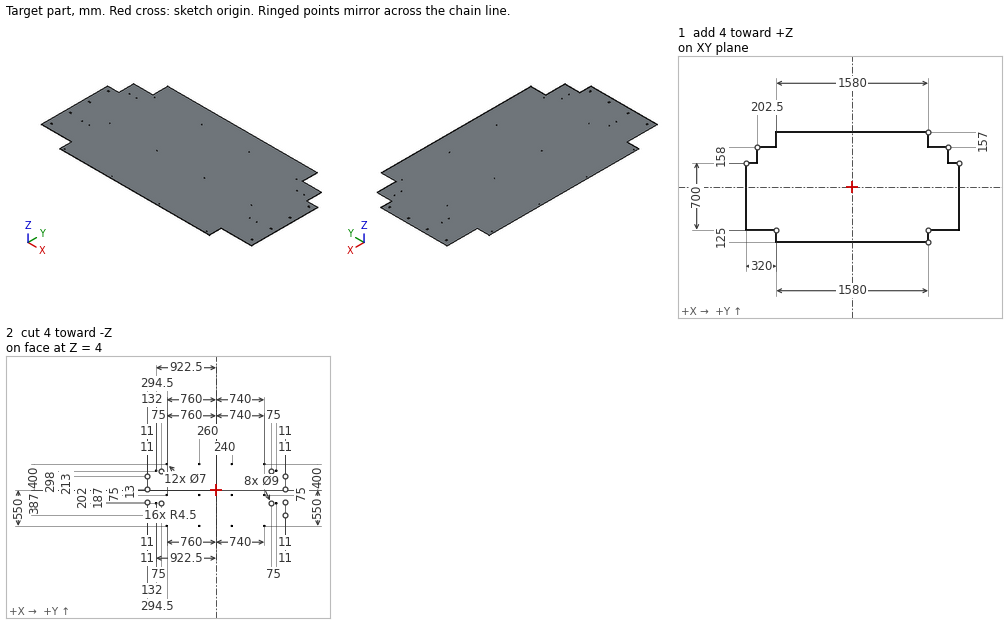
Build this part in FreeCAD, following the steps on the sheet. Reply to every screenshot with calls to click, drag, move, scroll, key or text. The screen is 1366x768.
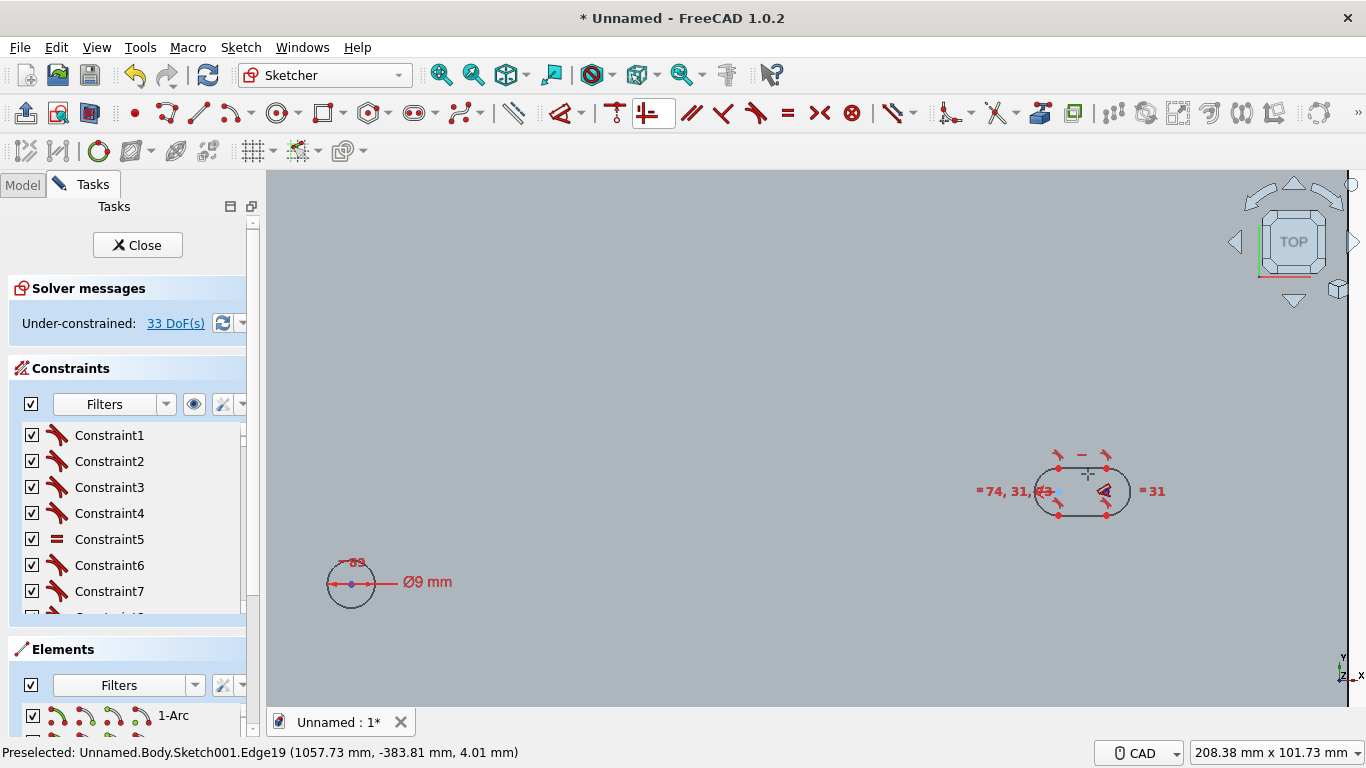
click(1073, 468)
click(1083, 502)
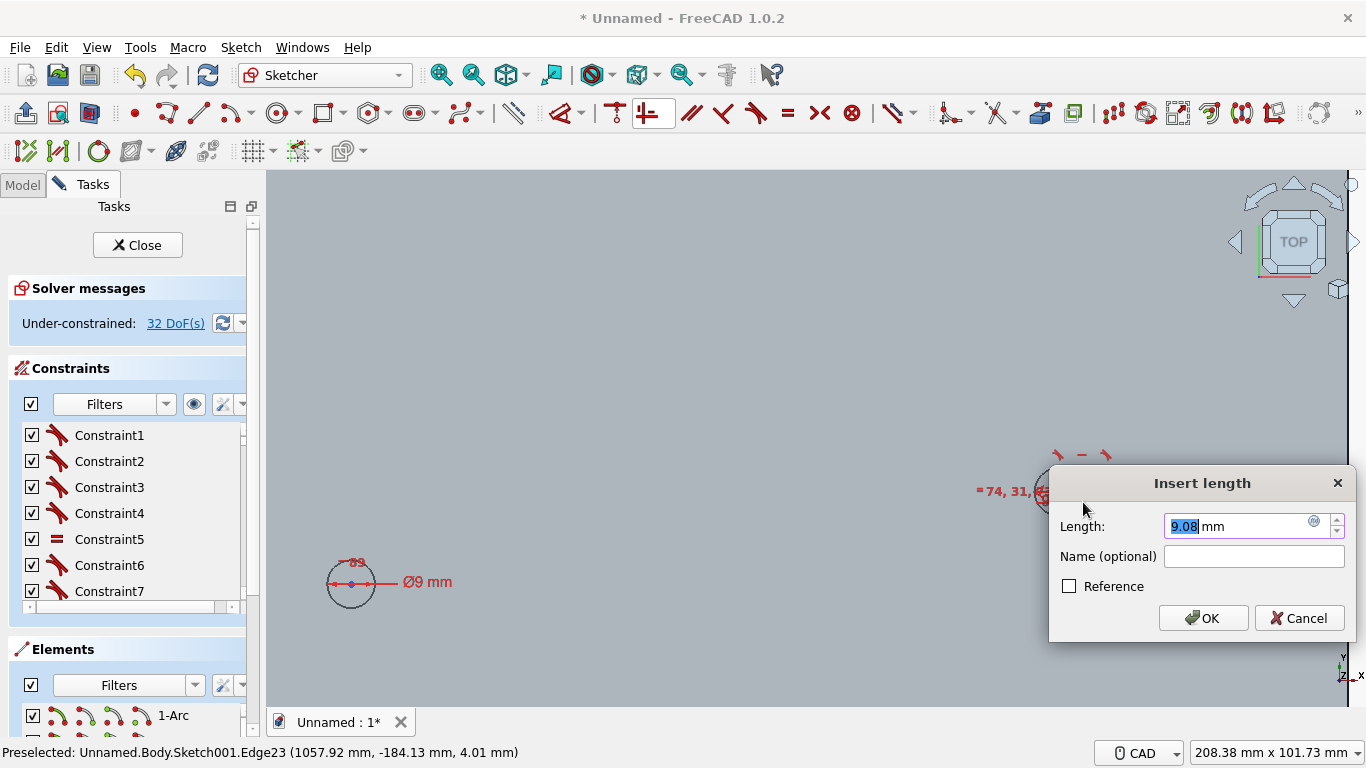
text(11)
key(Return)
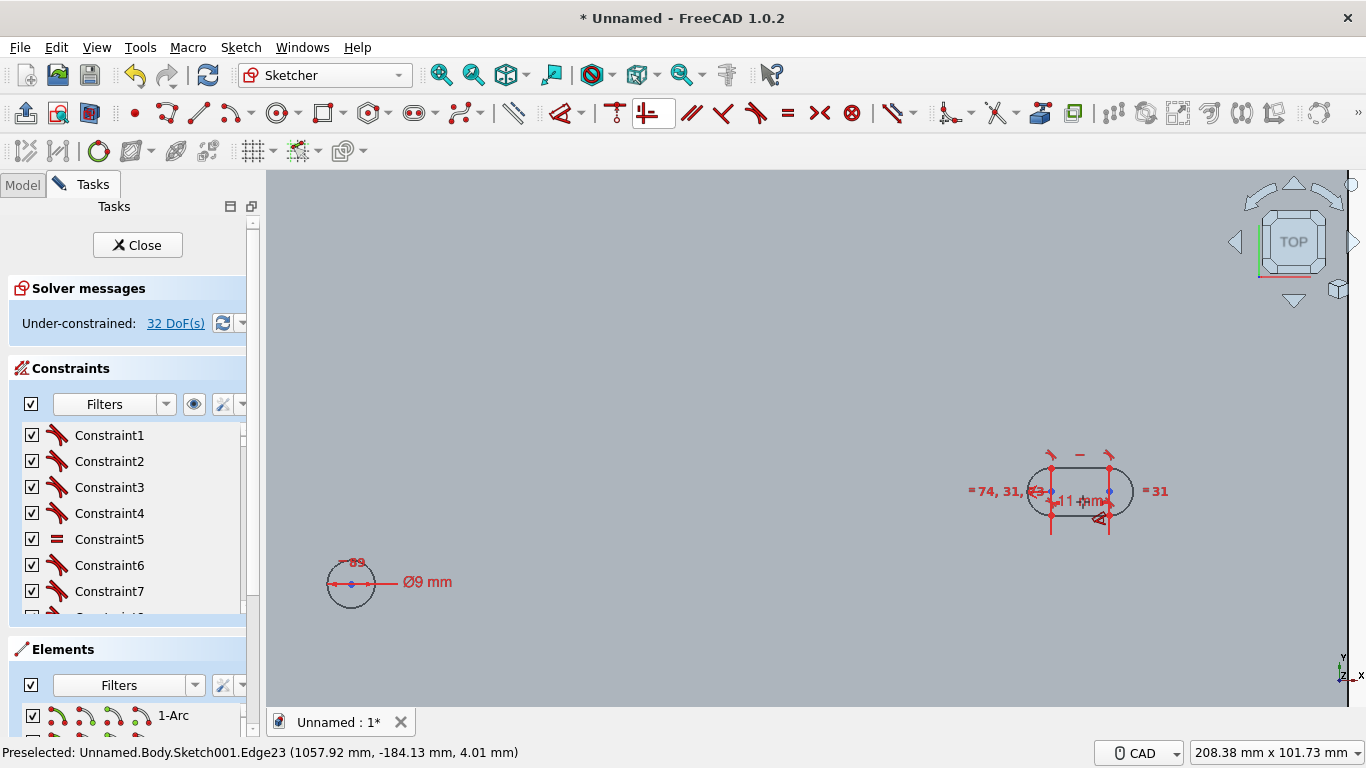
scroll(1088, 474, down, 14)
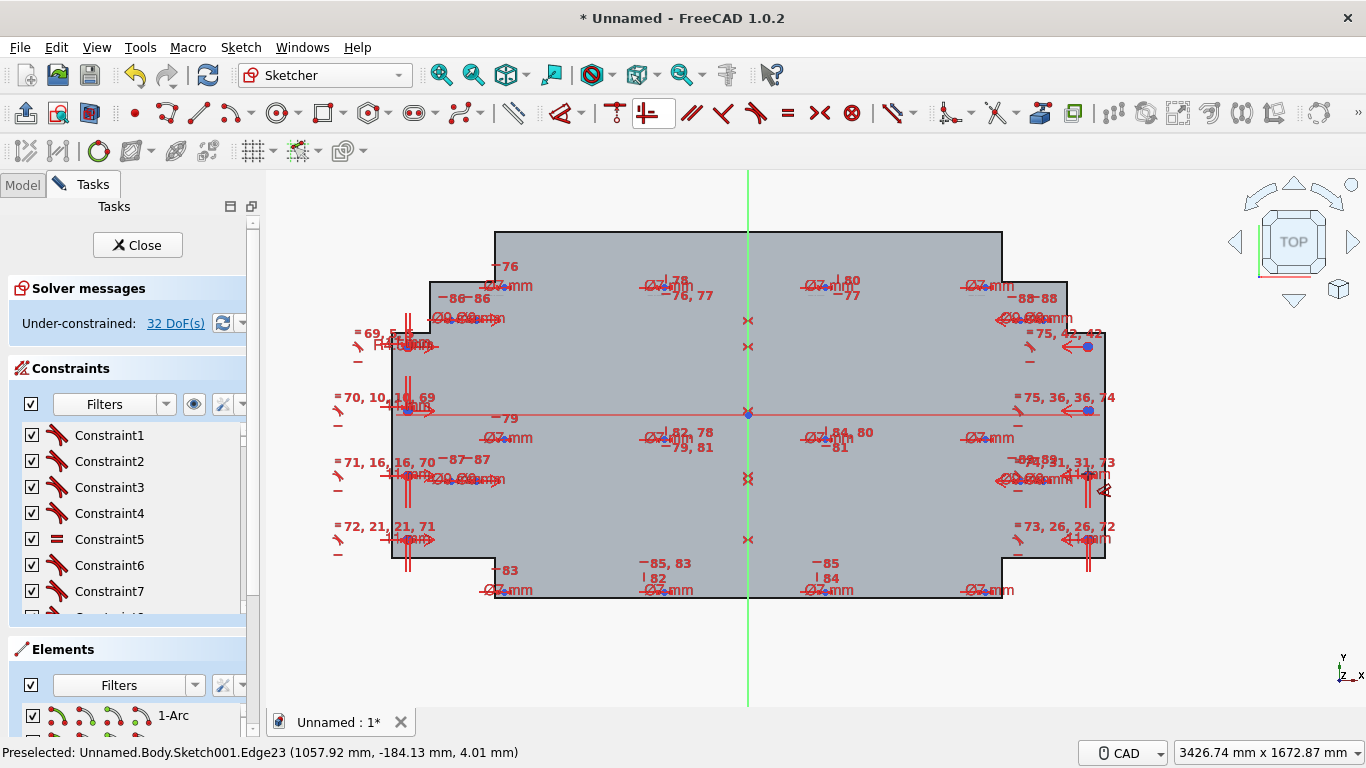
scroll(1088, 409, up, 13)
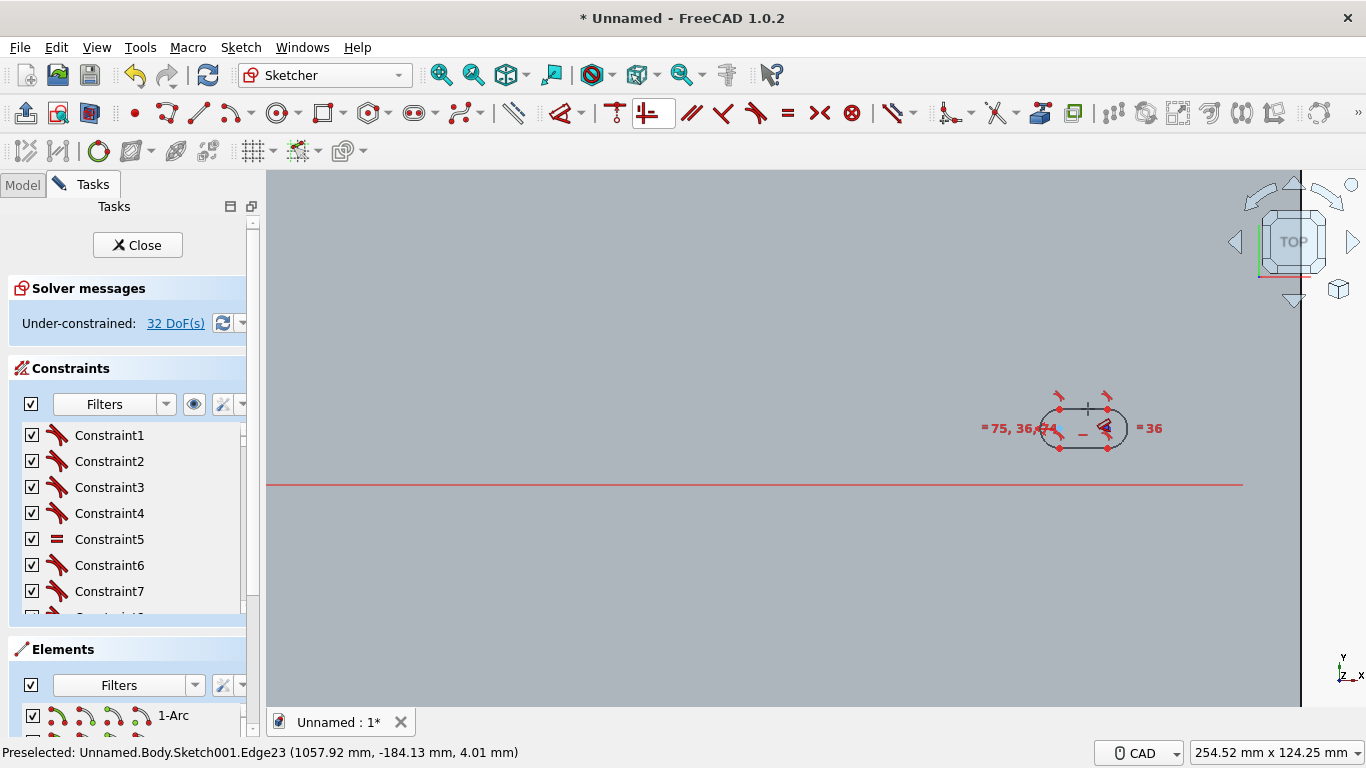
click(1074, 409)
click(1084, 375)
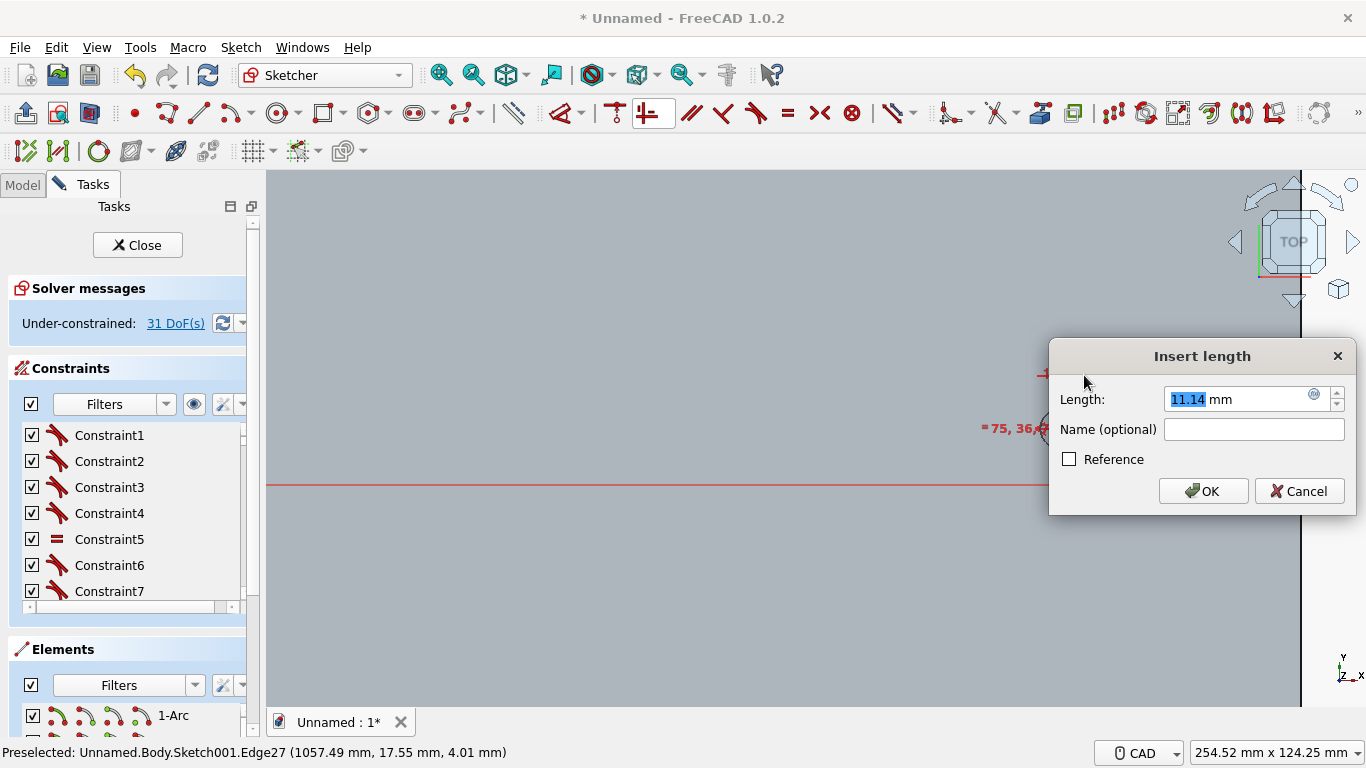
text(11)
key(Return)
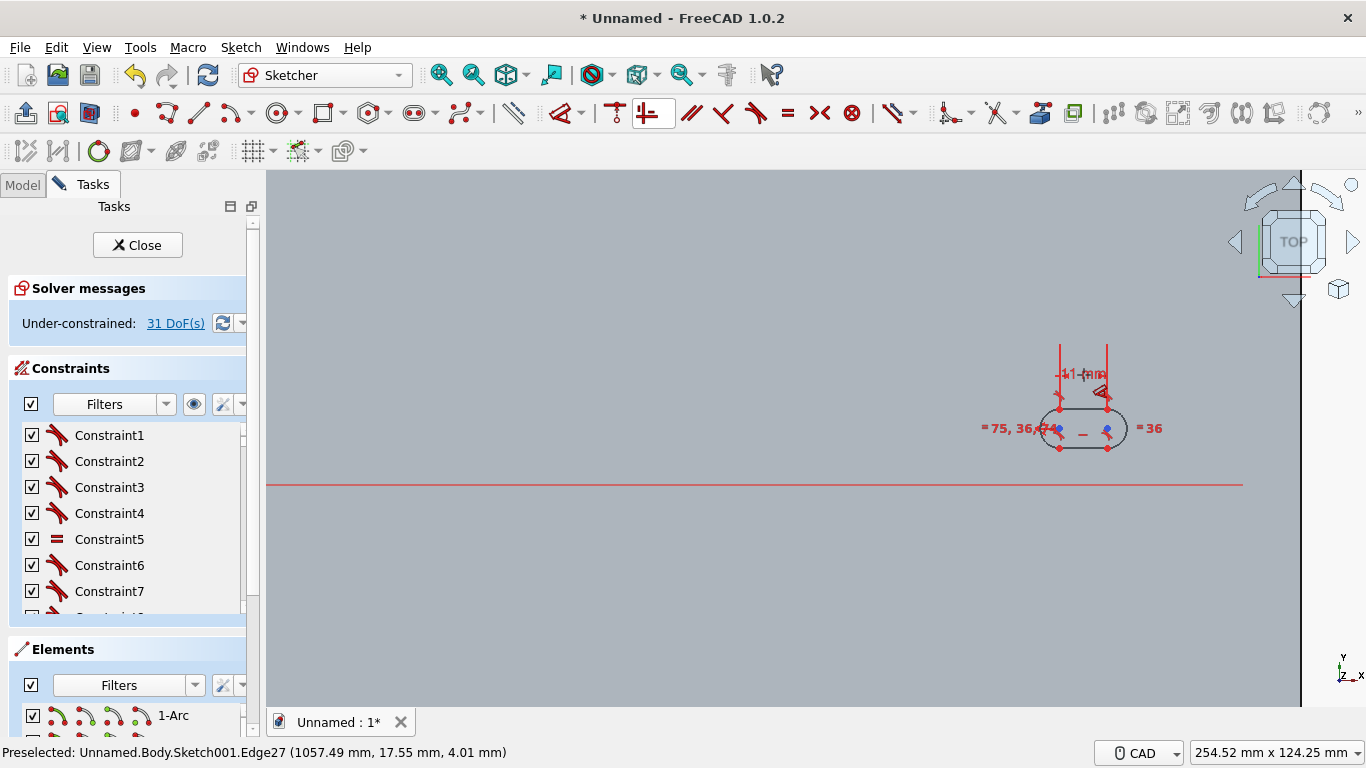
scroll(1088, 409, down, 13)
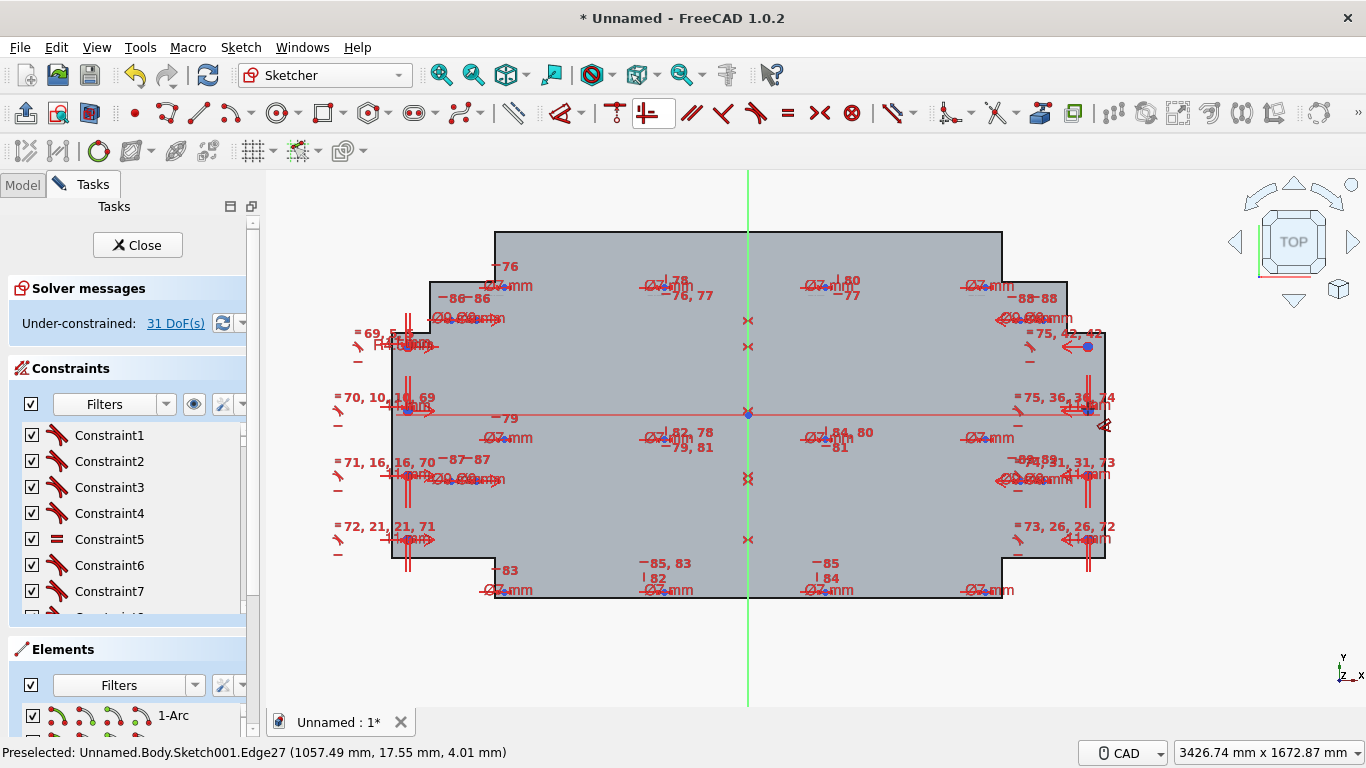
scroll(1088, 346, up, 14)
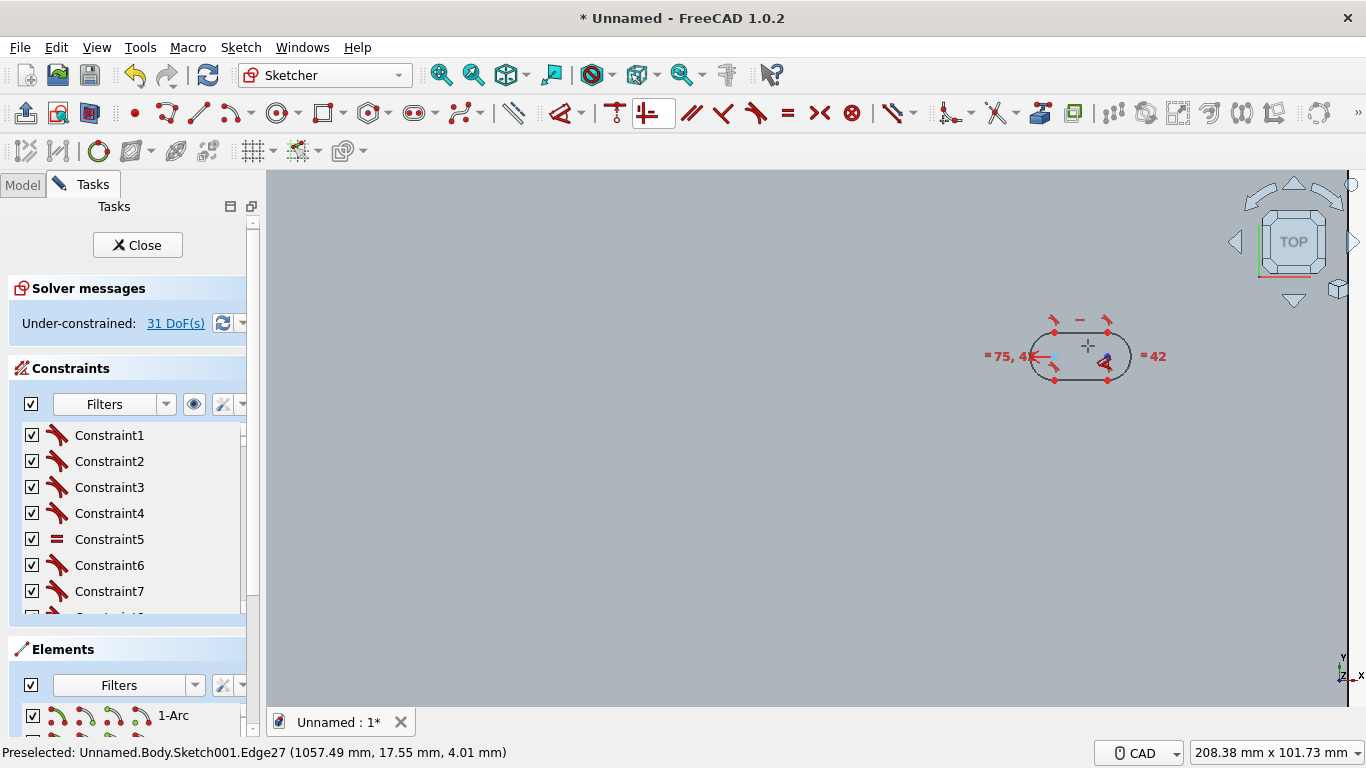
click(1070, 333)
click(1081, 299)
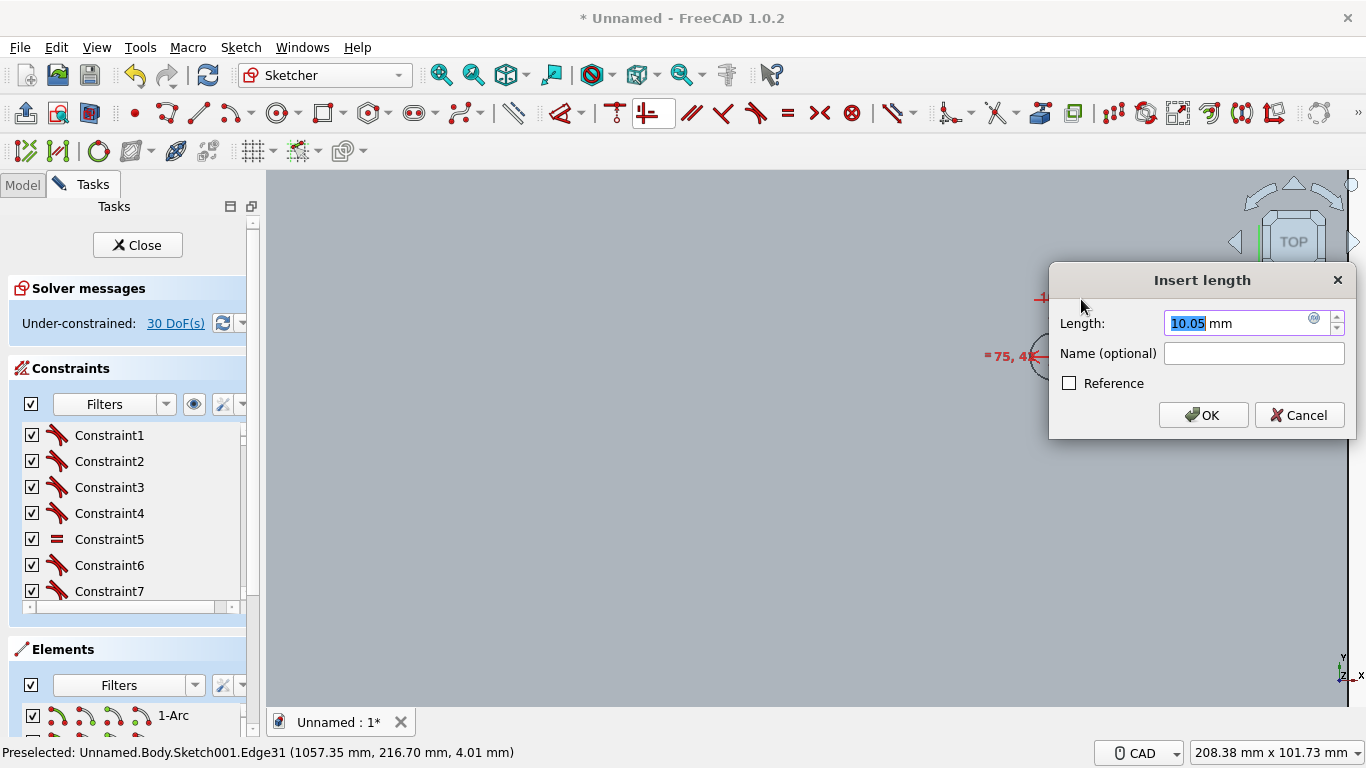
text(11)
key(Return)